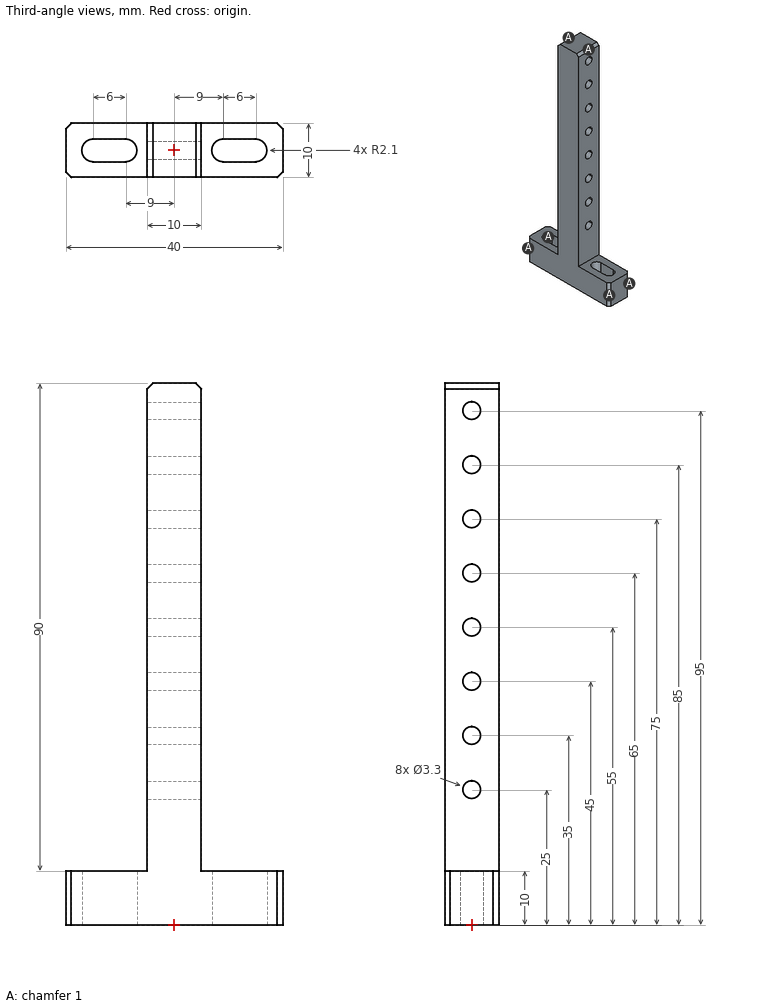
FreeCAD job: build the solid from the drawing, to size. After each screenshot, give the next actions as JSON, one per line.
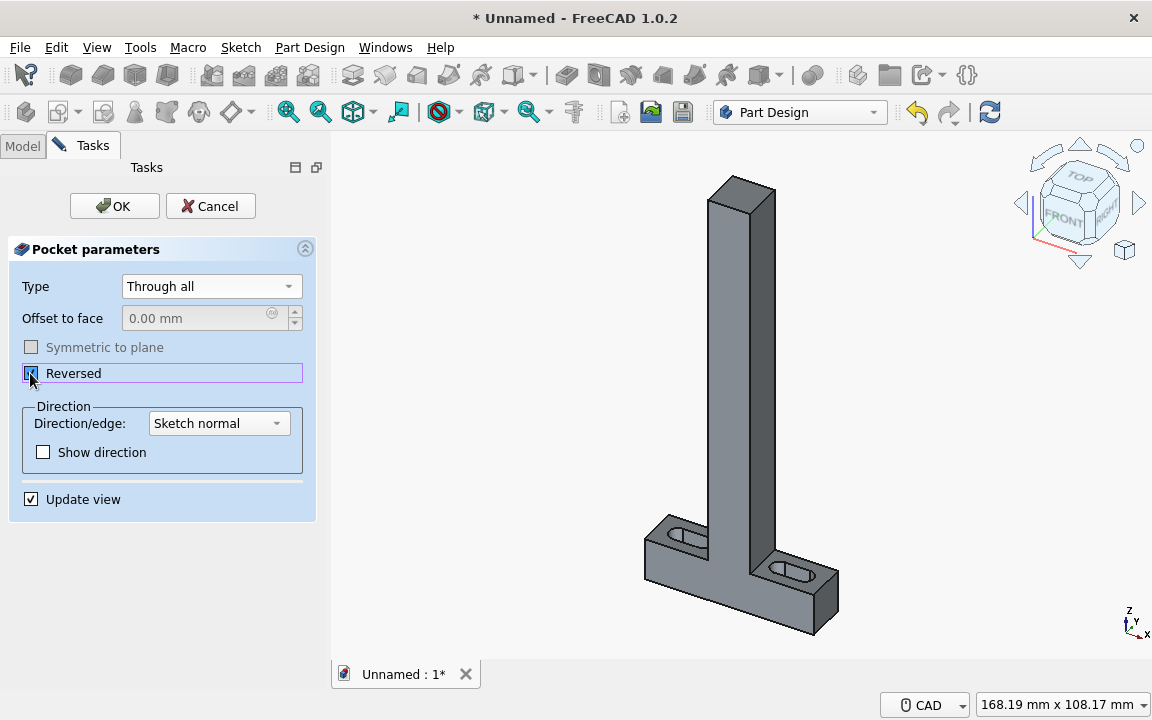
{"action": "left_click", "coordinate": [115, 206]}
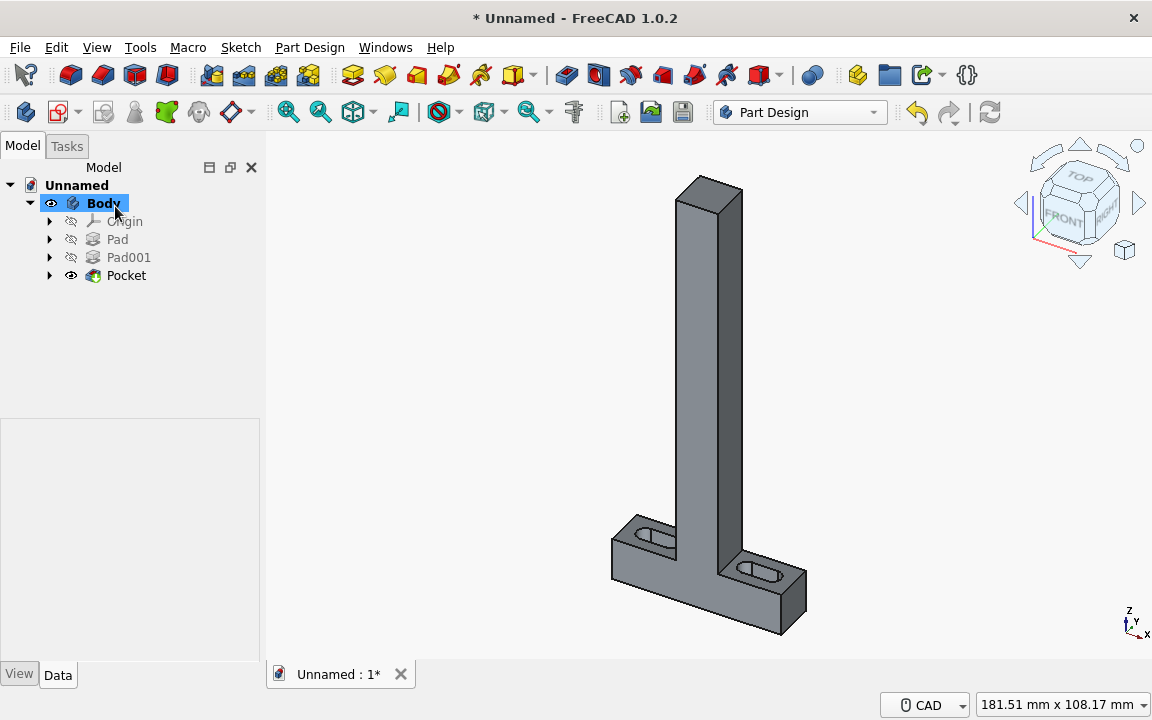
{"action": "left_click", "coordinate": [730, 227]}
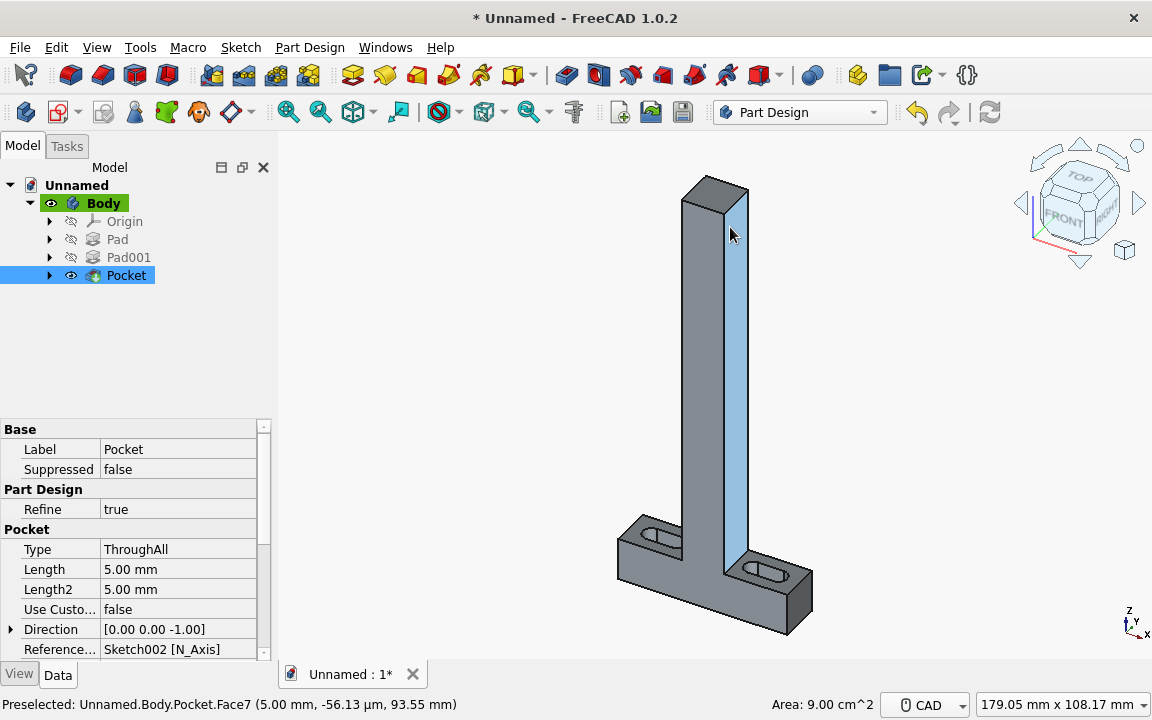
{"action": "left_click", "coordinate": [58, 112]}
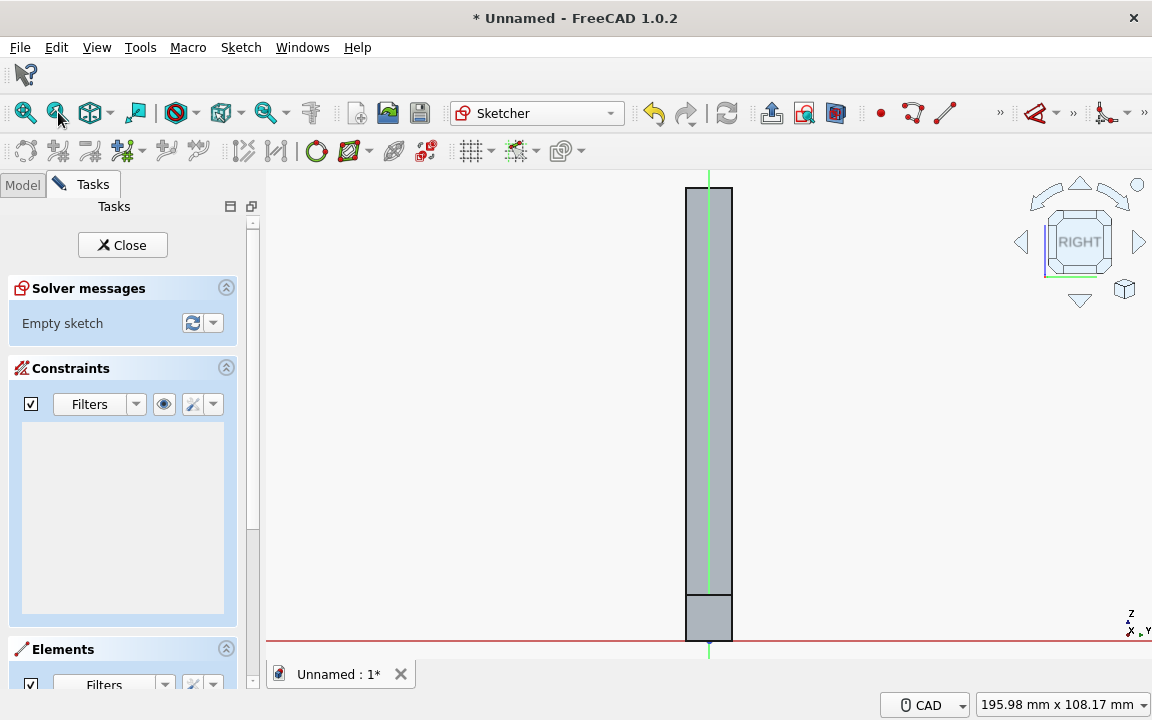
{"action": "scroll", "coordinate": [501, 399], "scroll_direction": "down", "scroll_amount": 2}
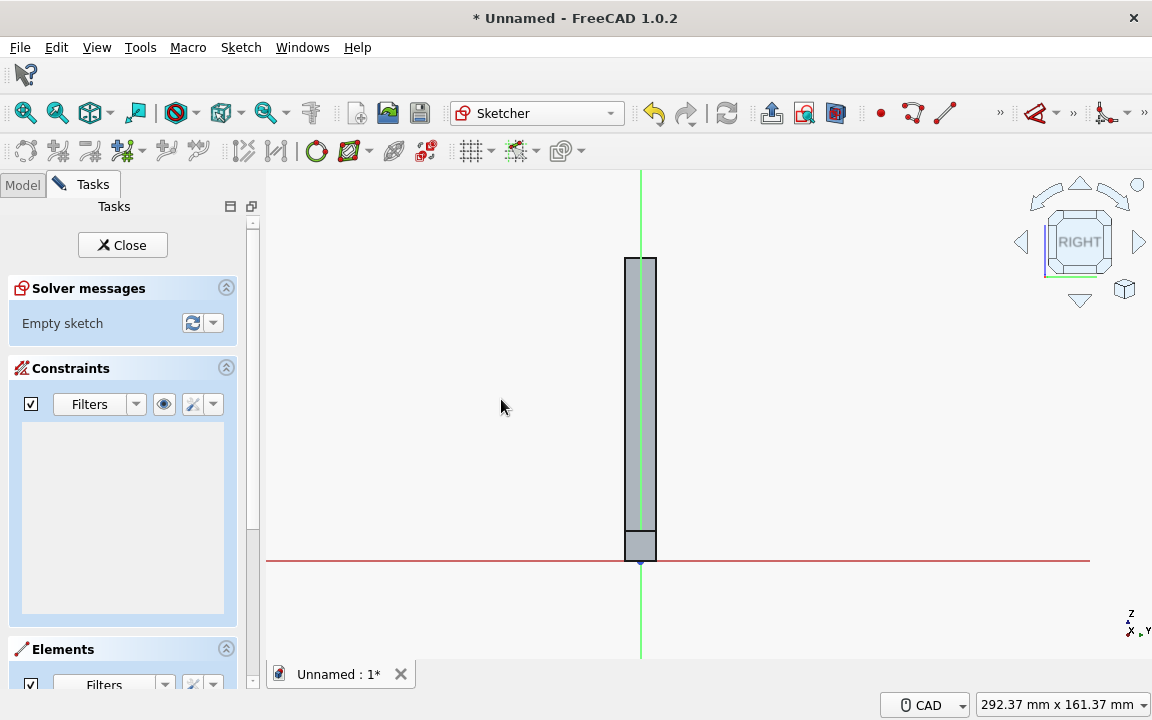
{"action": "key", "text": "g c"}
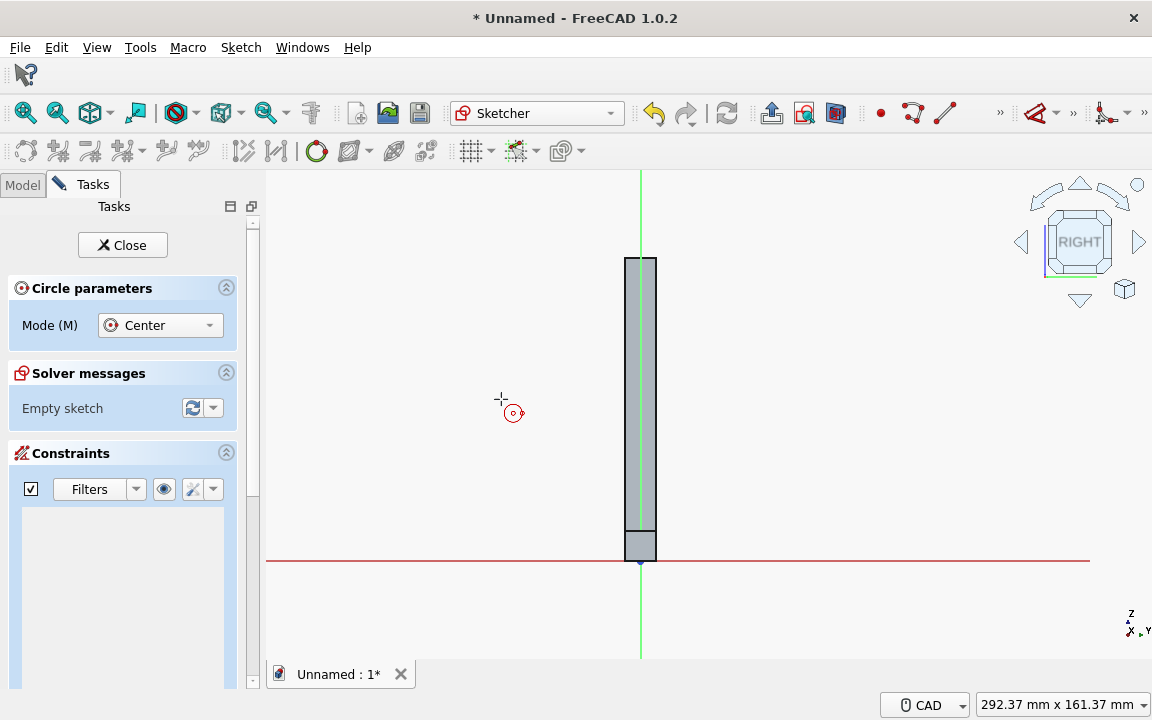
{"action": "scroll", "coordinate": [641, 485], "scroll_direction": "up", "scroll_amount": 8}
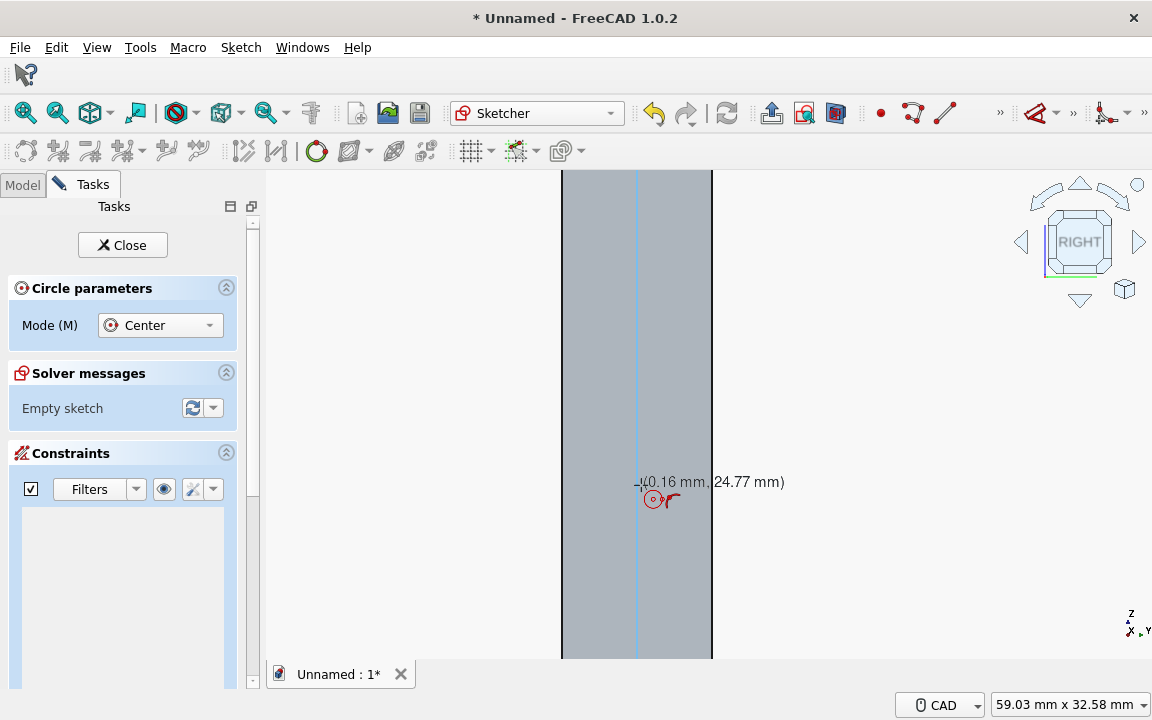
{"action": "scroll", "coordinate": [641, 485], "scroll_direction": "down", "scroll_amount": 8}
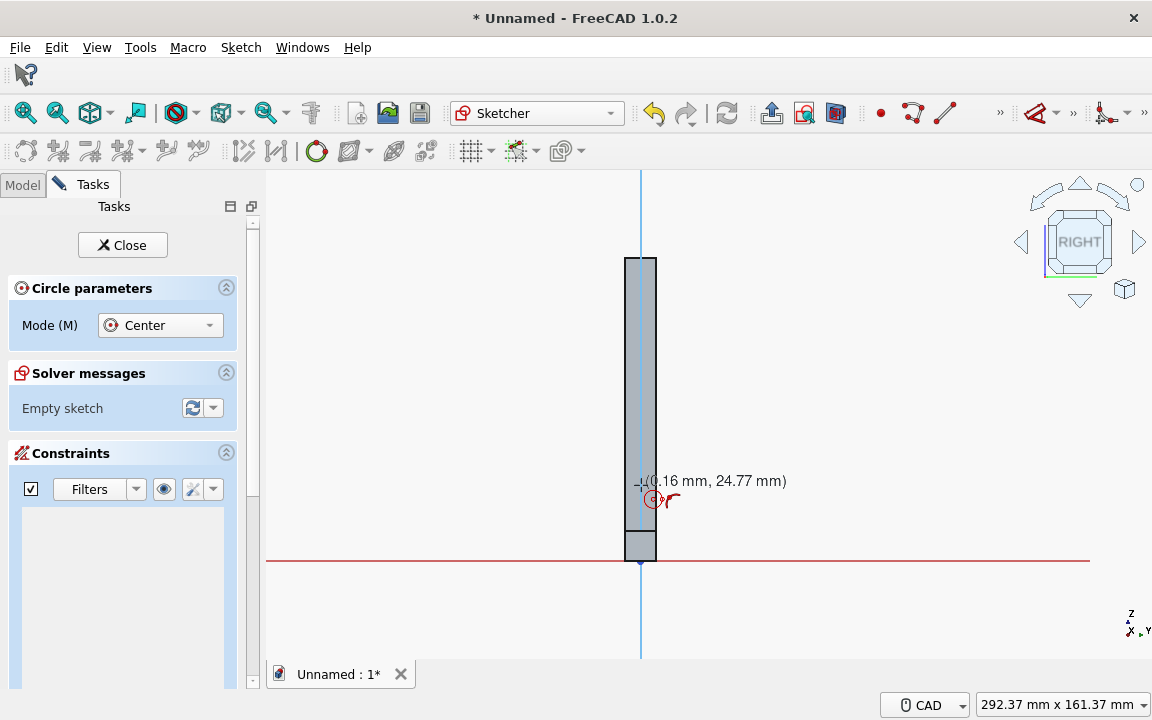
{"action": "left_click", "coordinate": [641, 485]}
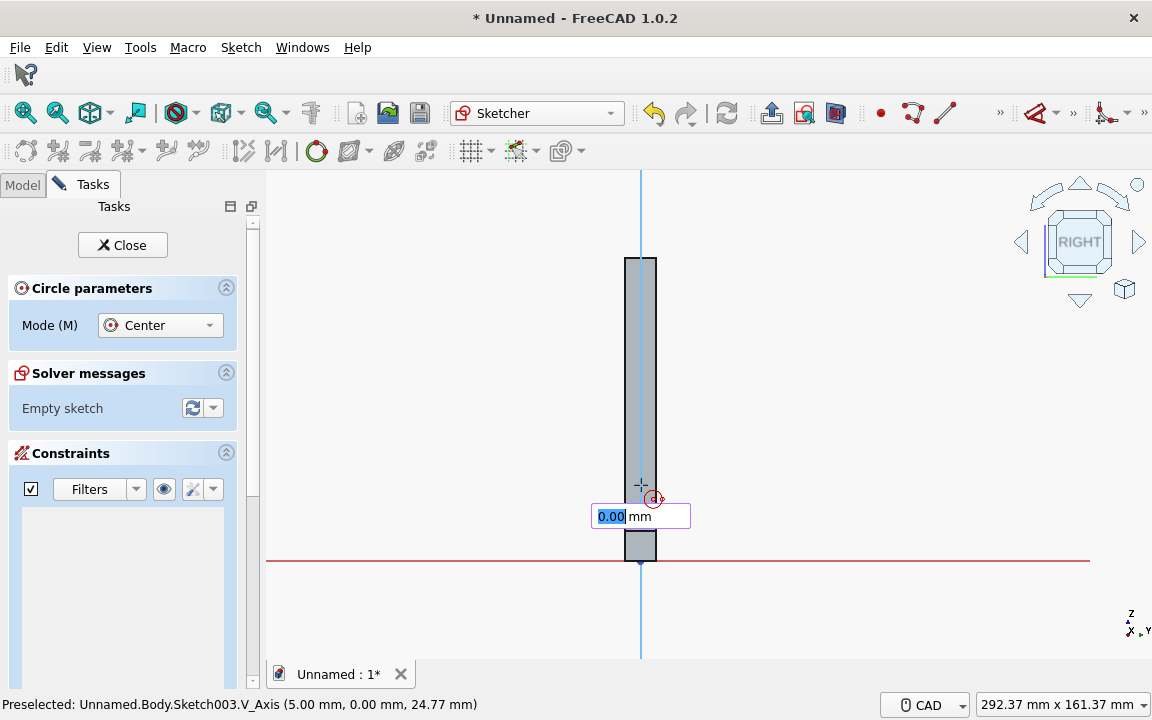
{"action": "scroll", "coordinate": [645, 484], "scroll_direction": "up", "scroll_amount": 7}
{"action": "mouse_move", "coordinate": [645, 480]}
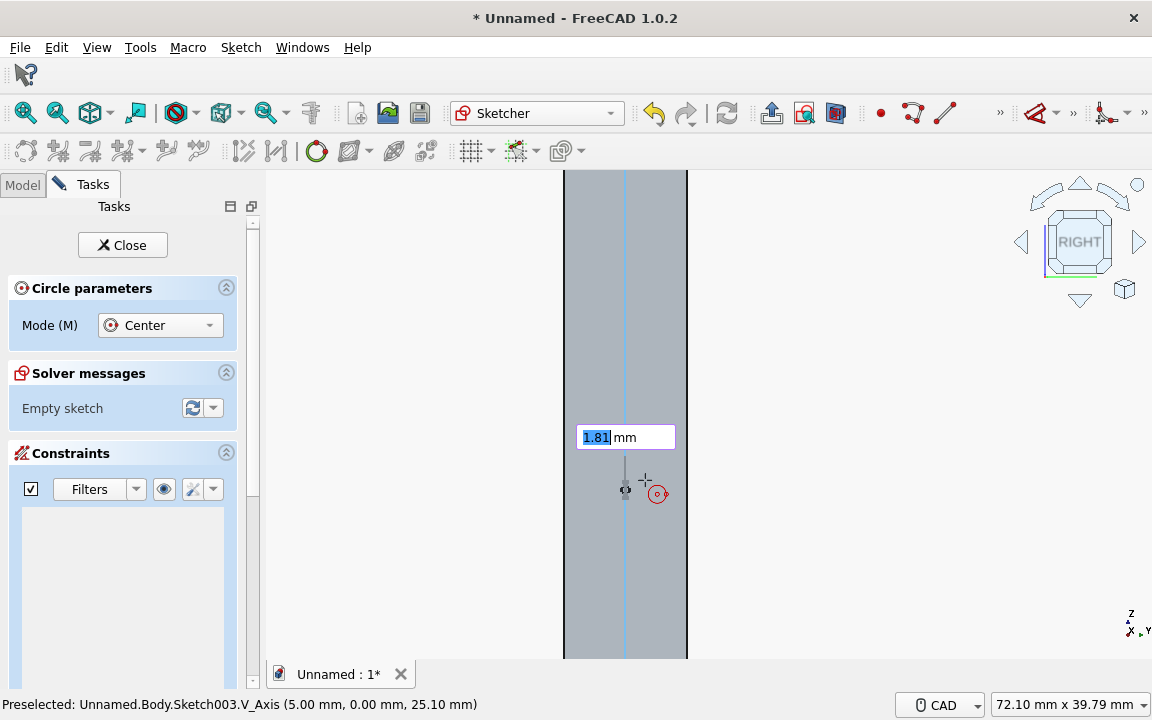
{"action": "type", "text": "3.3"}
{"action": "key", "text": "Return"}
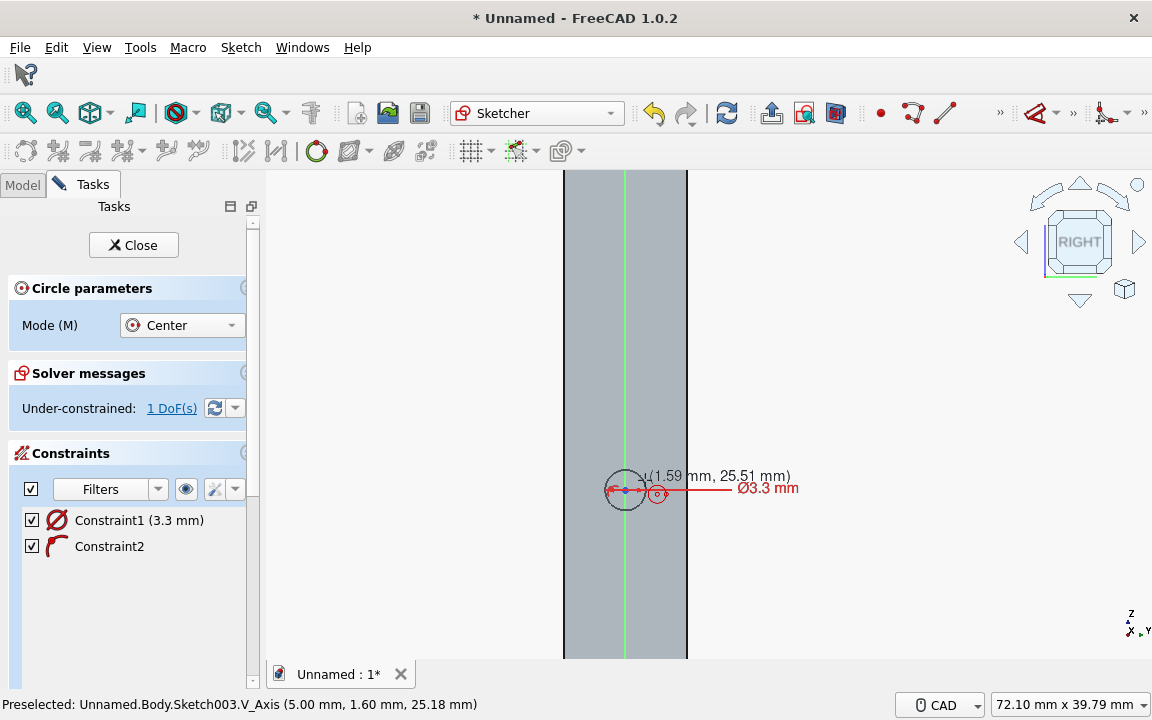
{"action": "scroll", "coordinate": [645, 484], "scroll_direction": "down", "scroll_amount": 7}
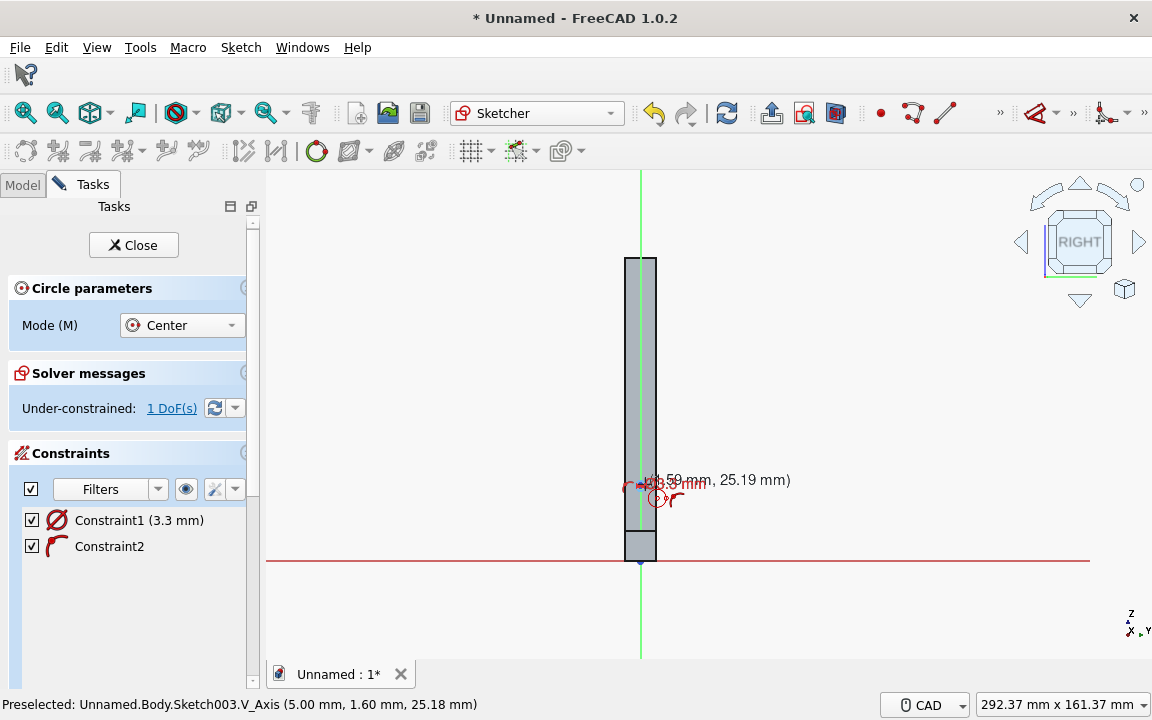
{"action": "left_click", "coordinate": [641, 455]}